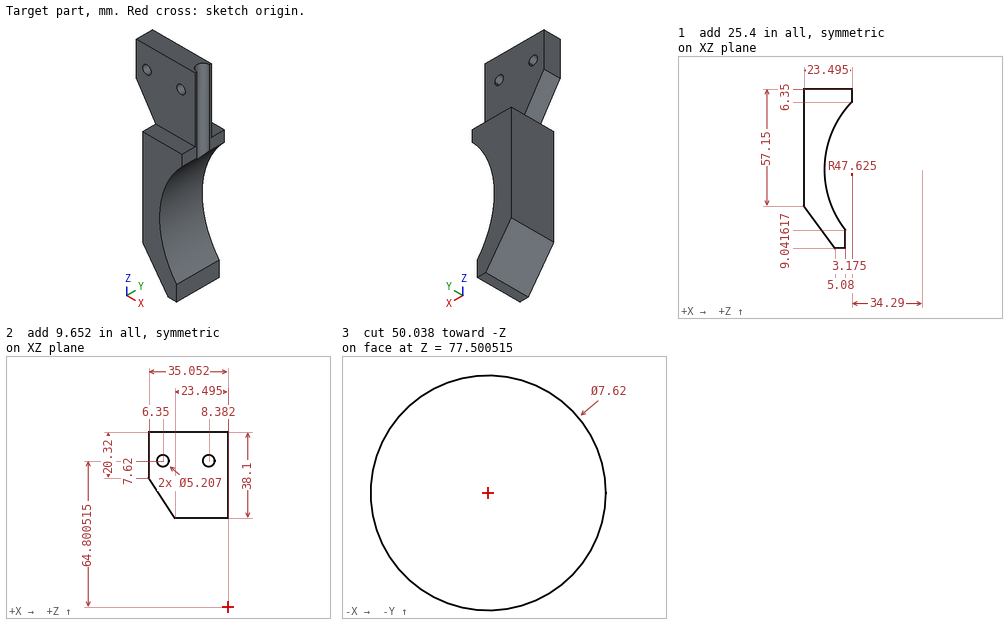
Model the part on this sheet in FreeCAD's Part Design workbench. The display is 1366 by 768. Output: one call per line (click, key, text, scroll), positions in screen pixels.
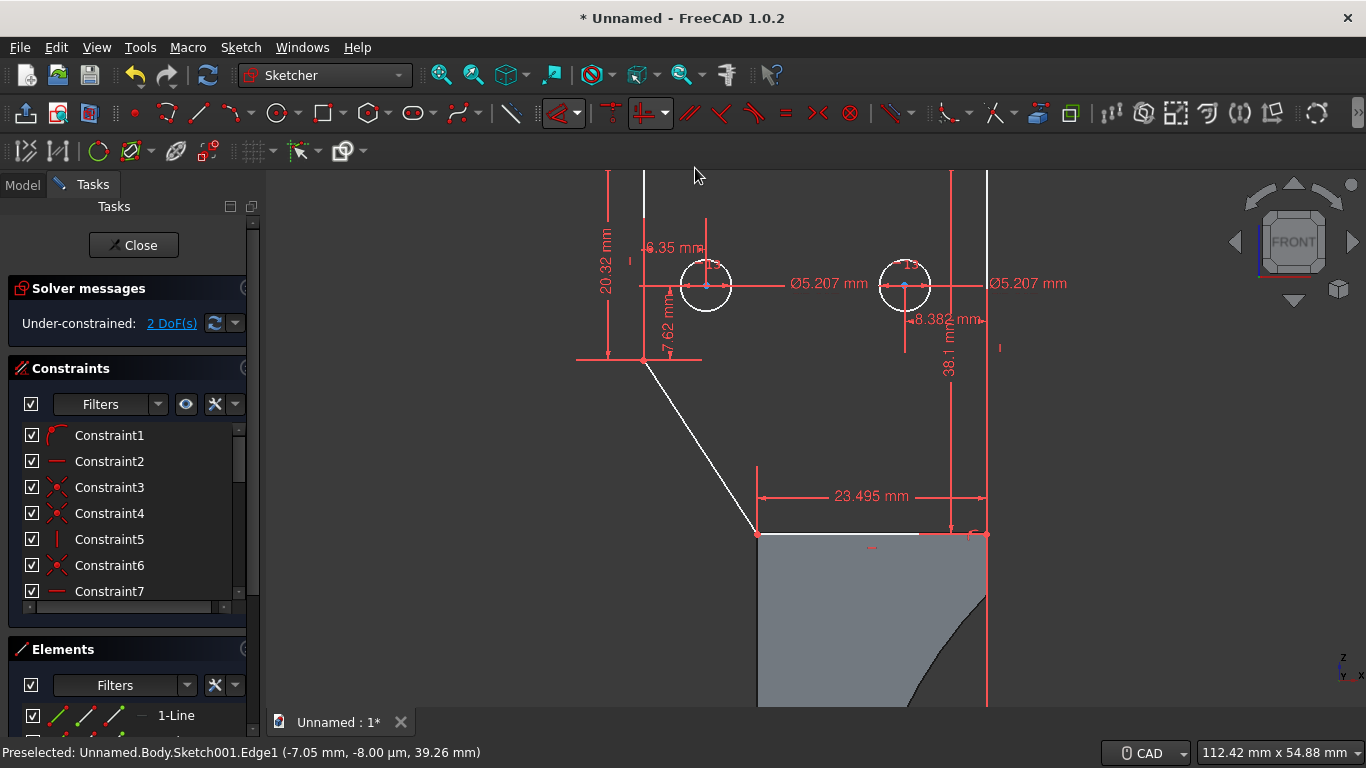
scroll(692, 356, down, 4)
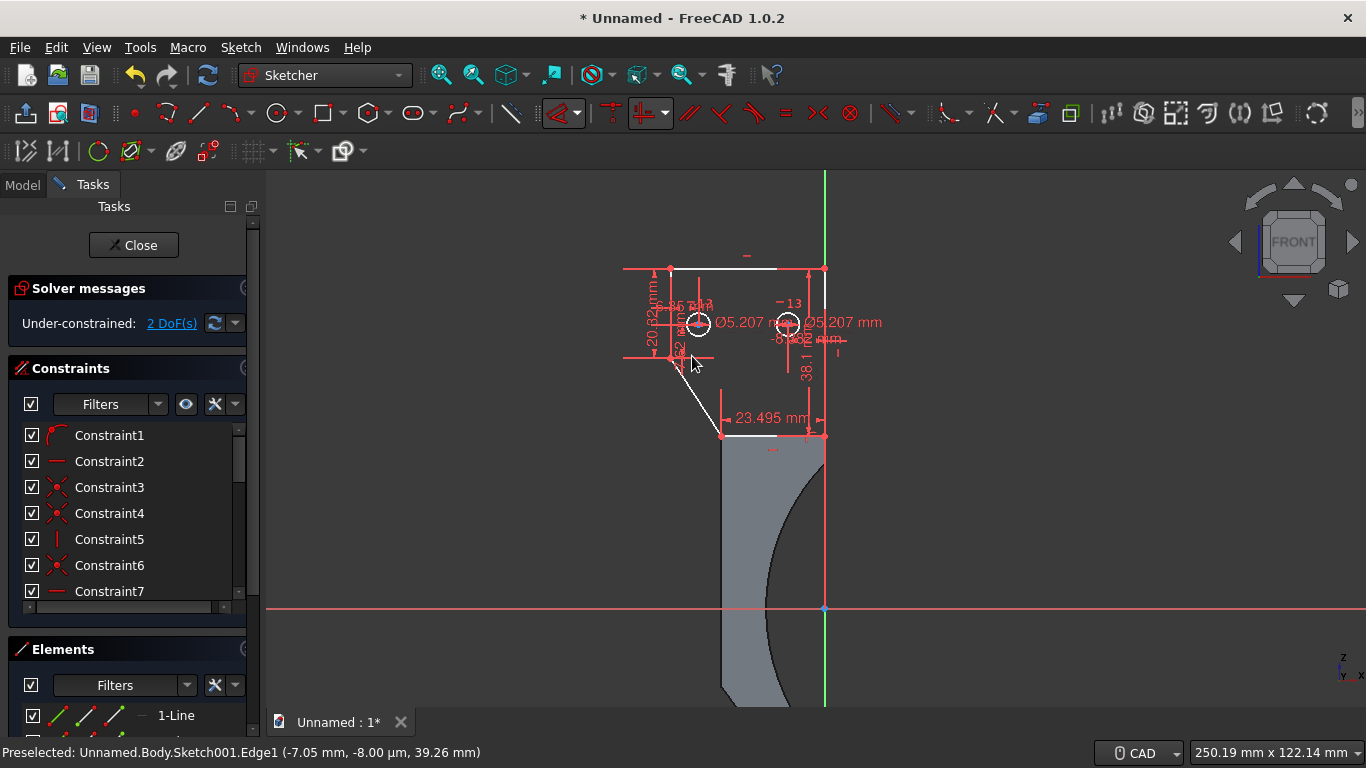
click(717, 269)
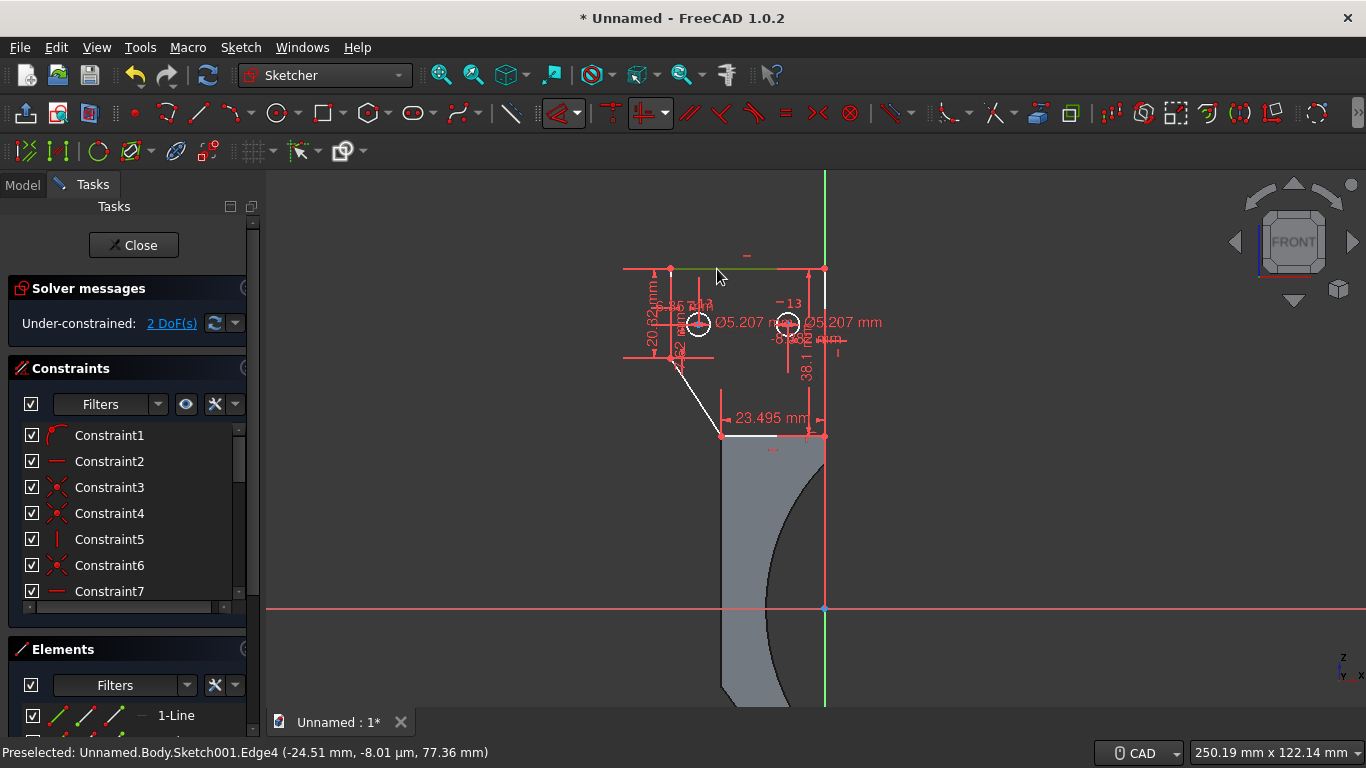
click(580, 114)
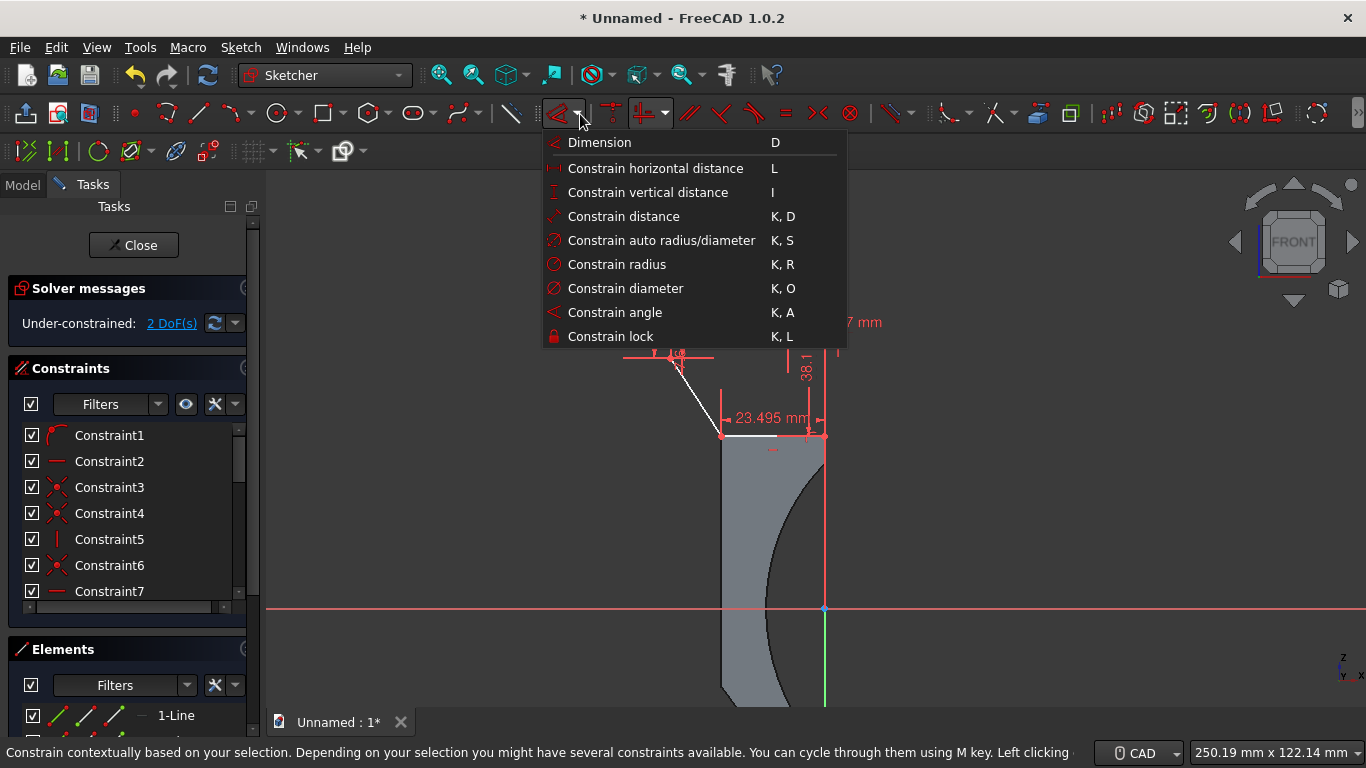
click(695, 168)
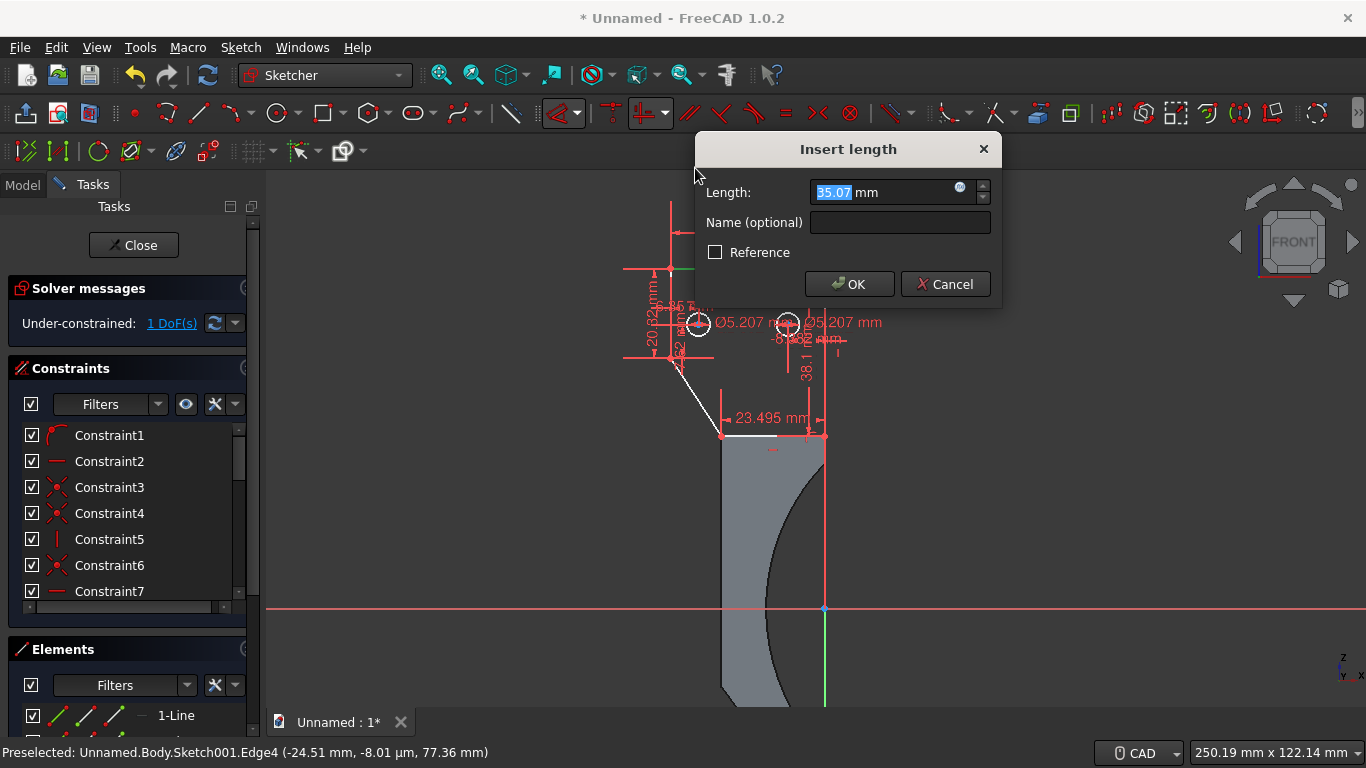
text(35.052)
key(Return)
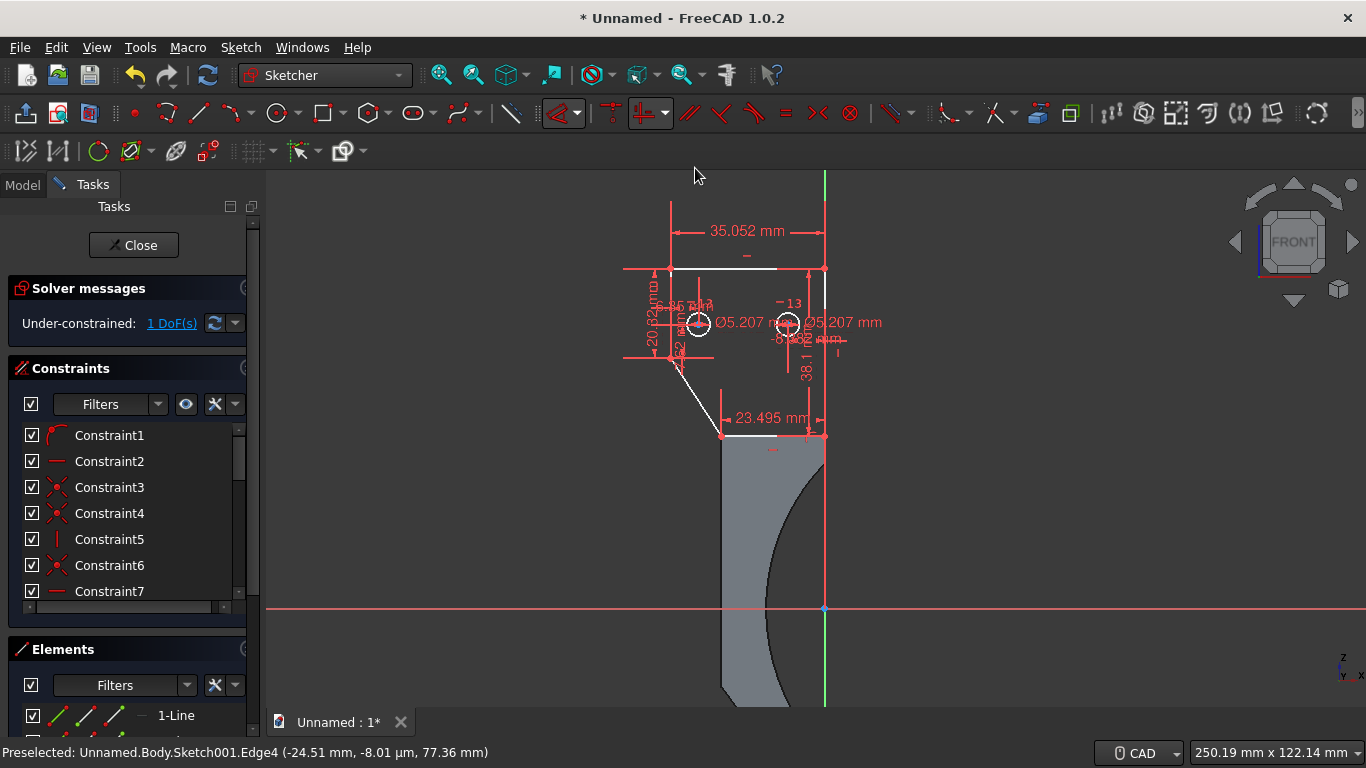
click(699, 325)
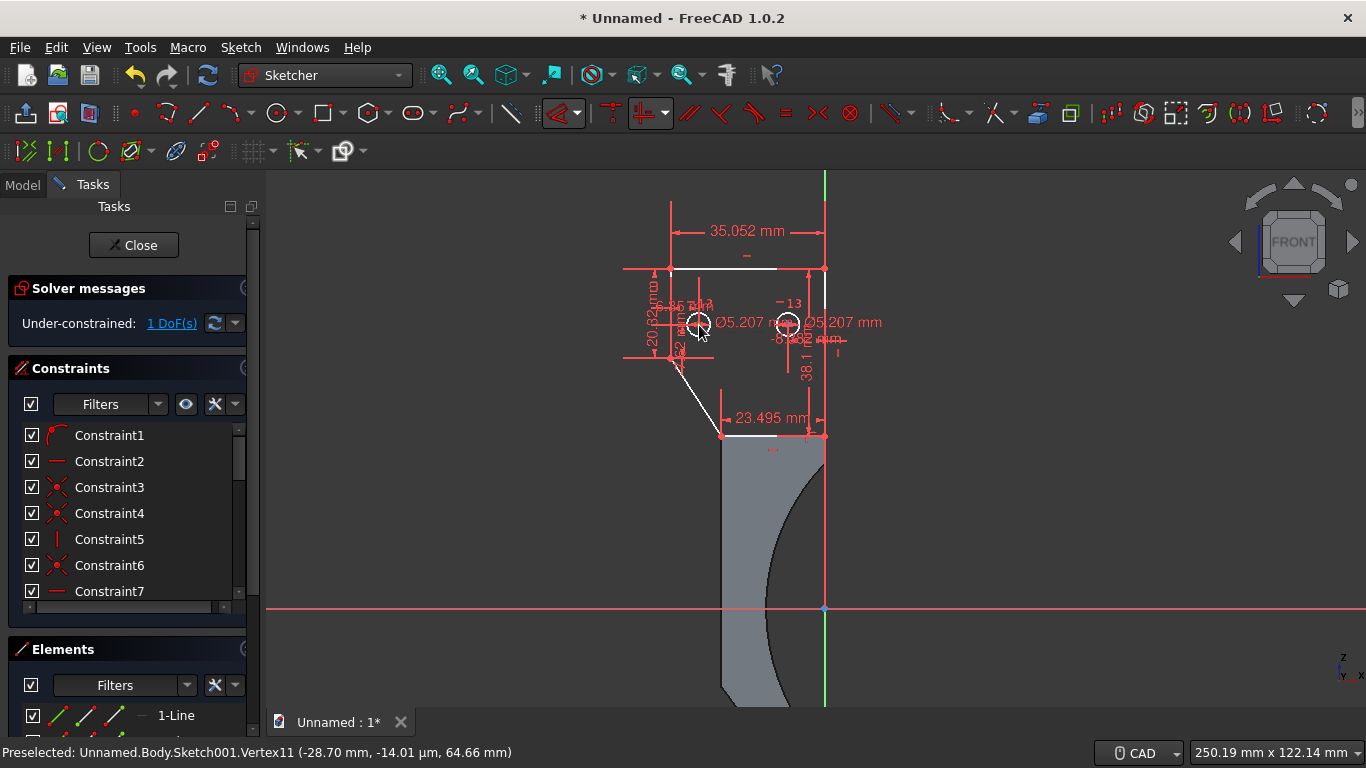
click(580, 114)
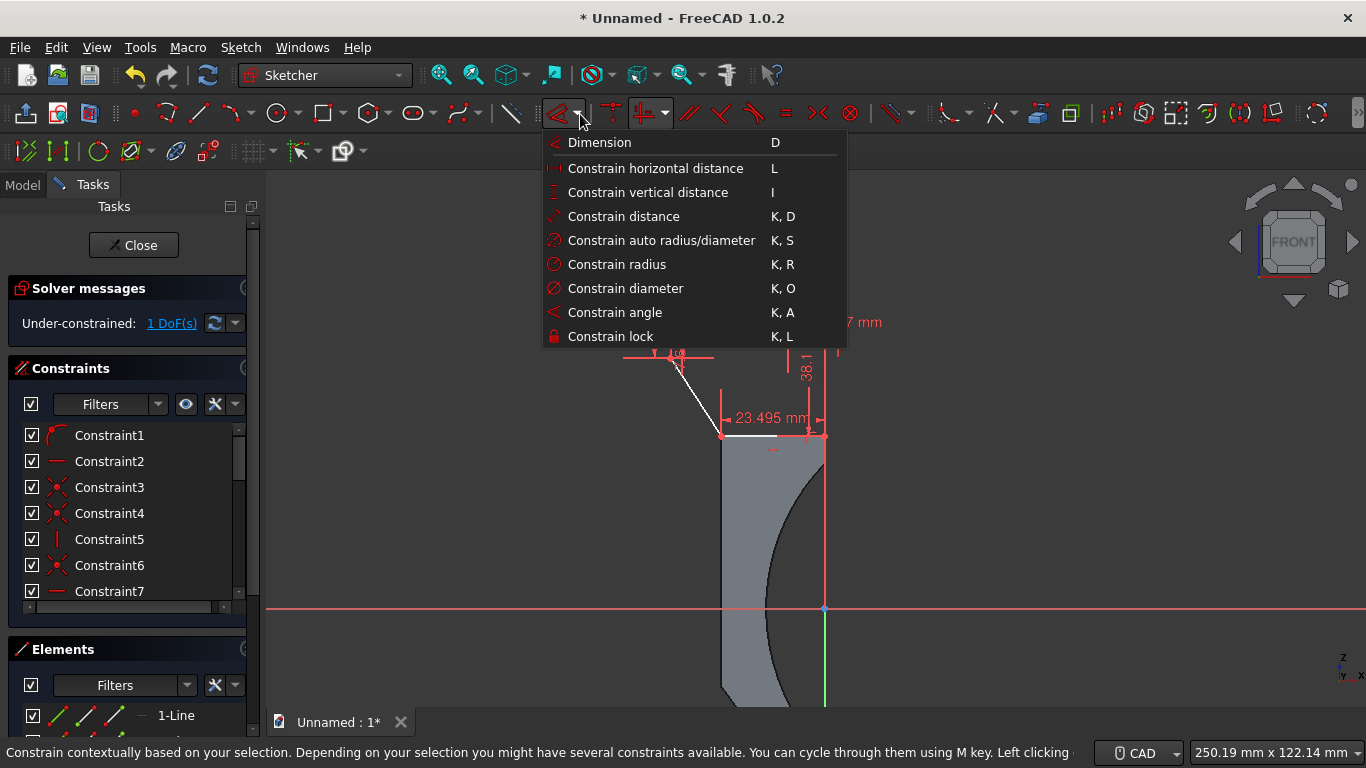
click(695, 192)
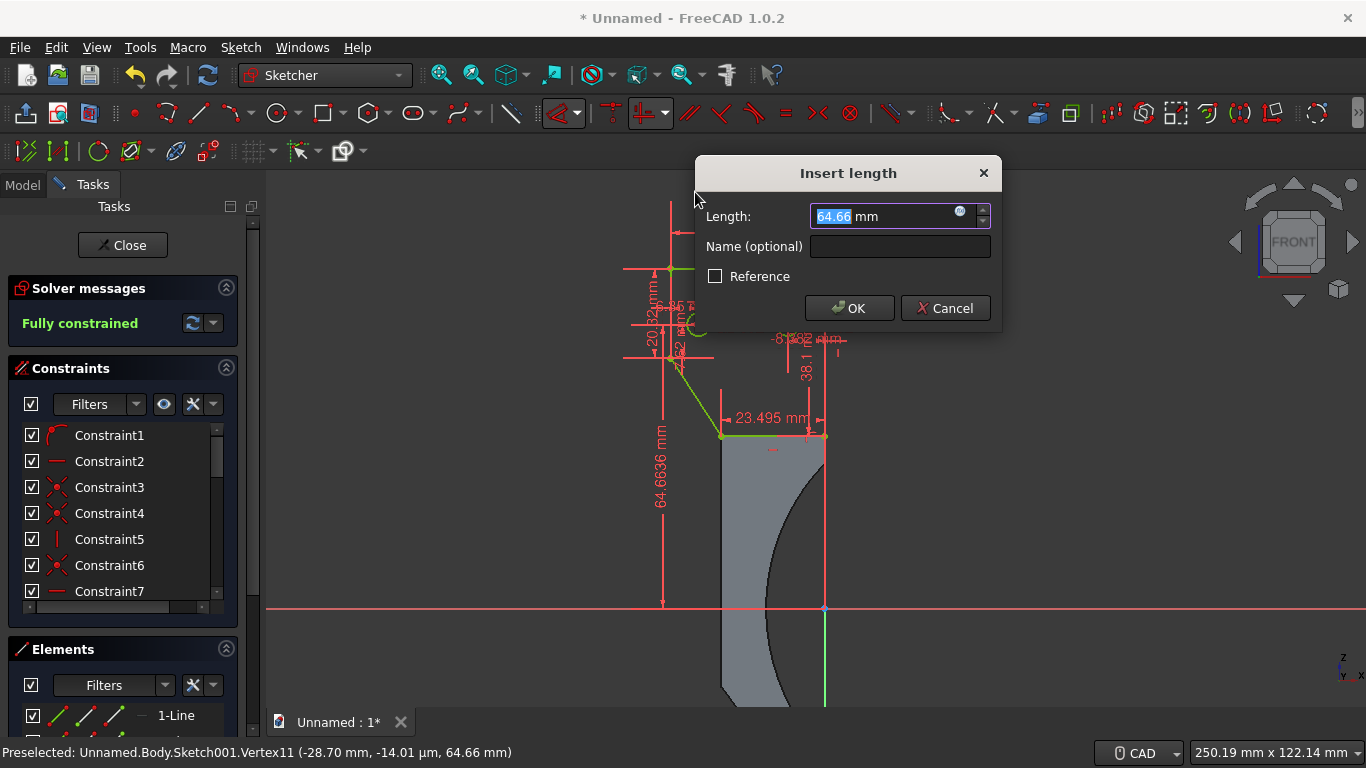
text(64.800515)
key(Return)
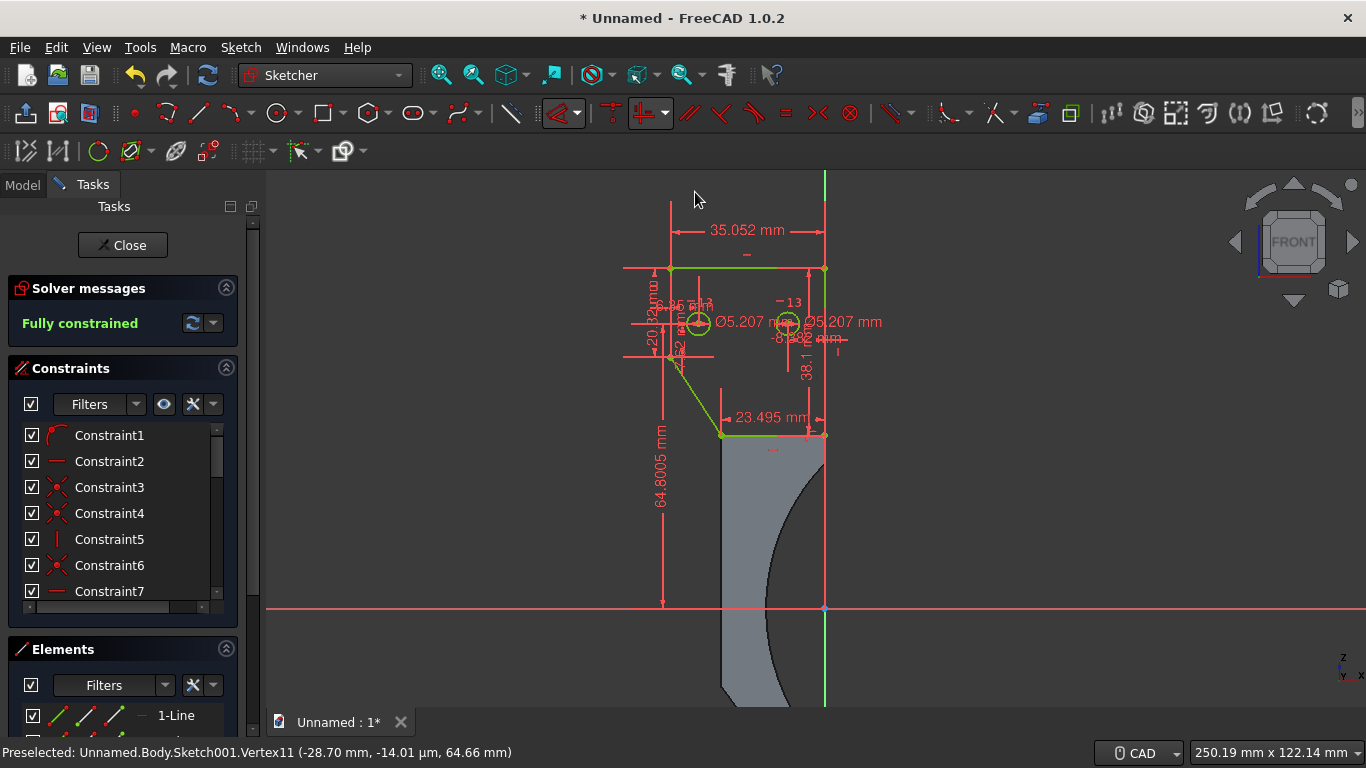
click(123, 245)